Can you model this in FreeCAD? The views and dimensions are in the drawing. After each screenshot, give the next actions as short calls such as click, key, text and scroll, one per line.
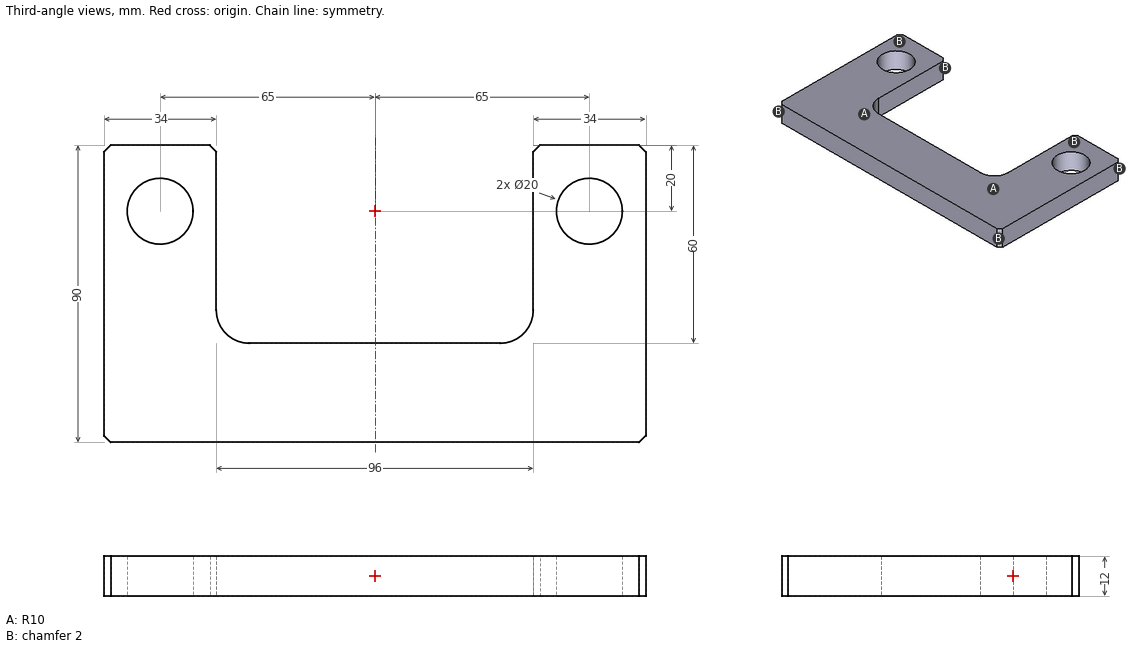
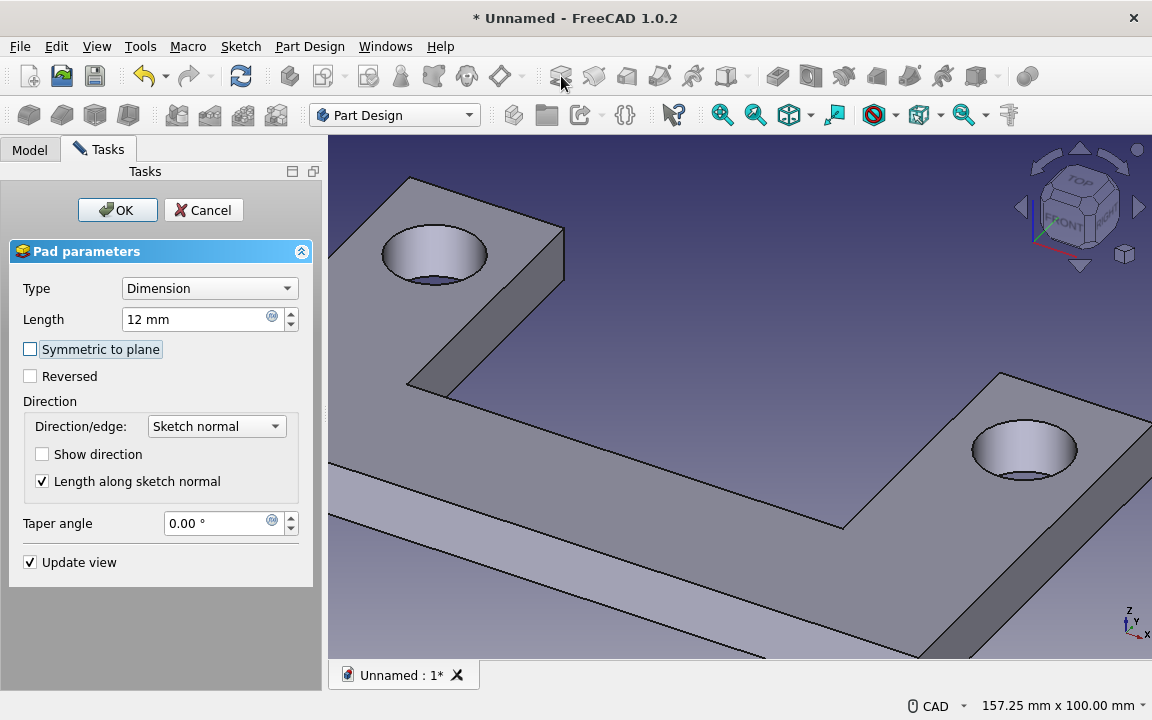
click(31, 349)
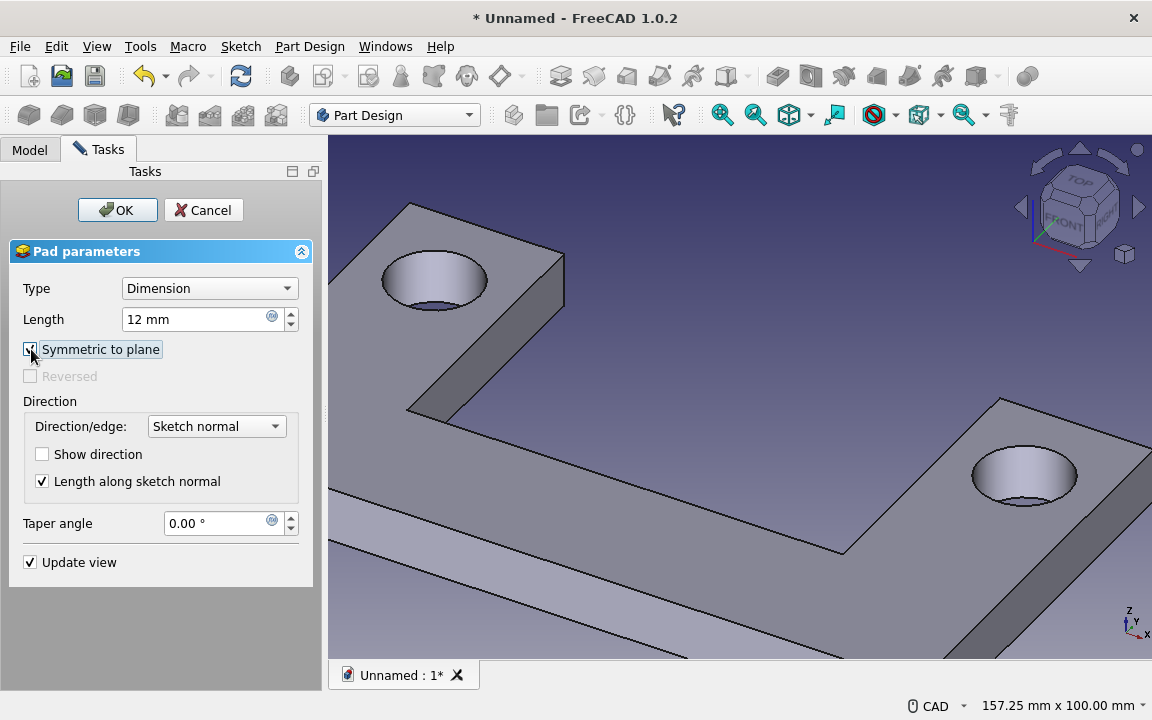
click(118, 210)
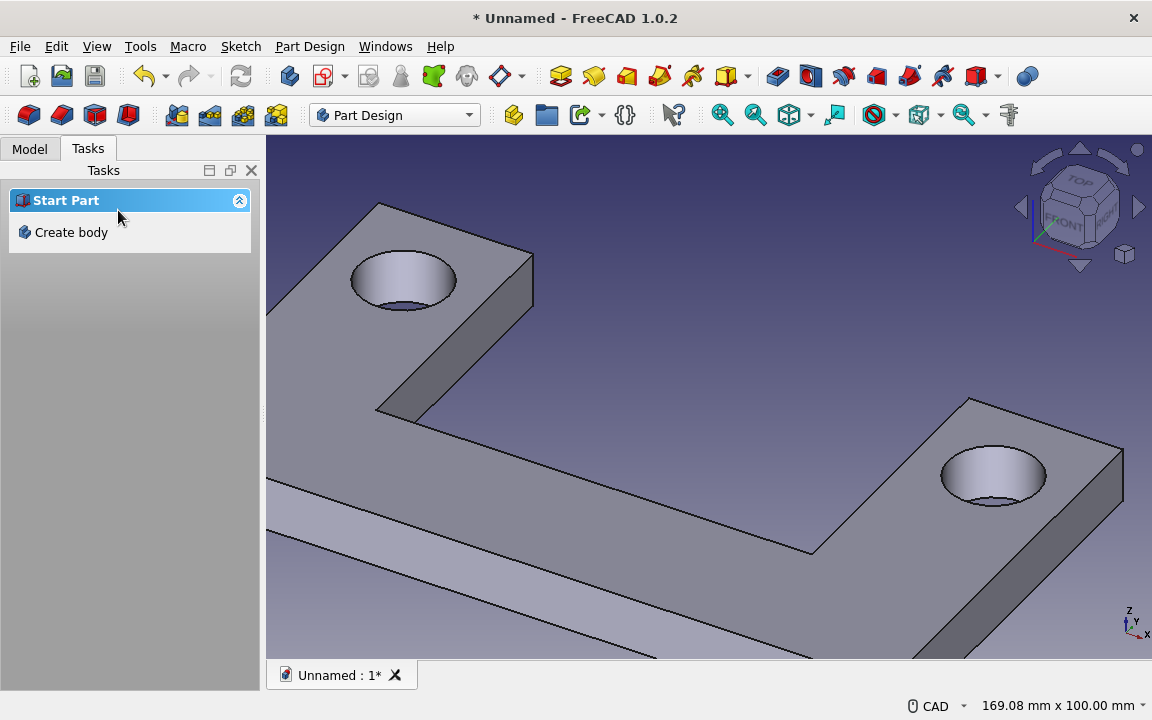
click(723, 116)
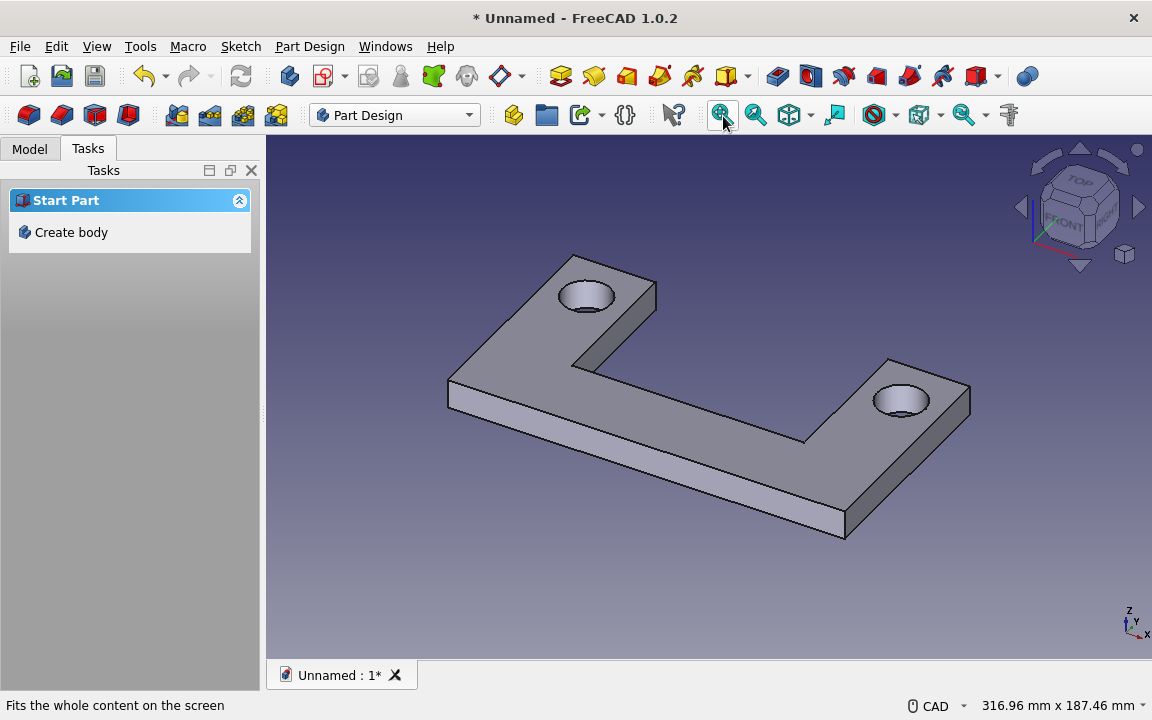
key(0)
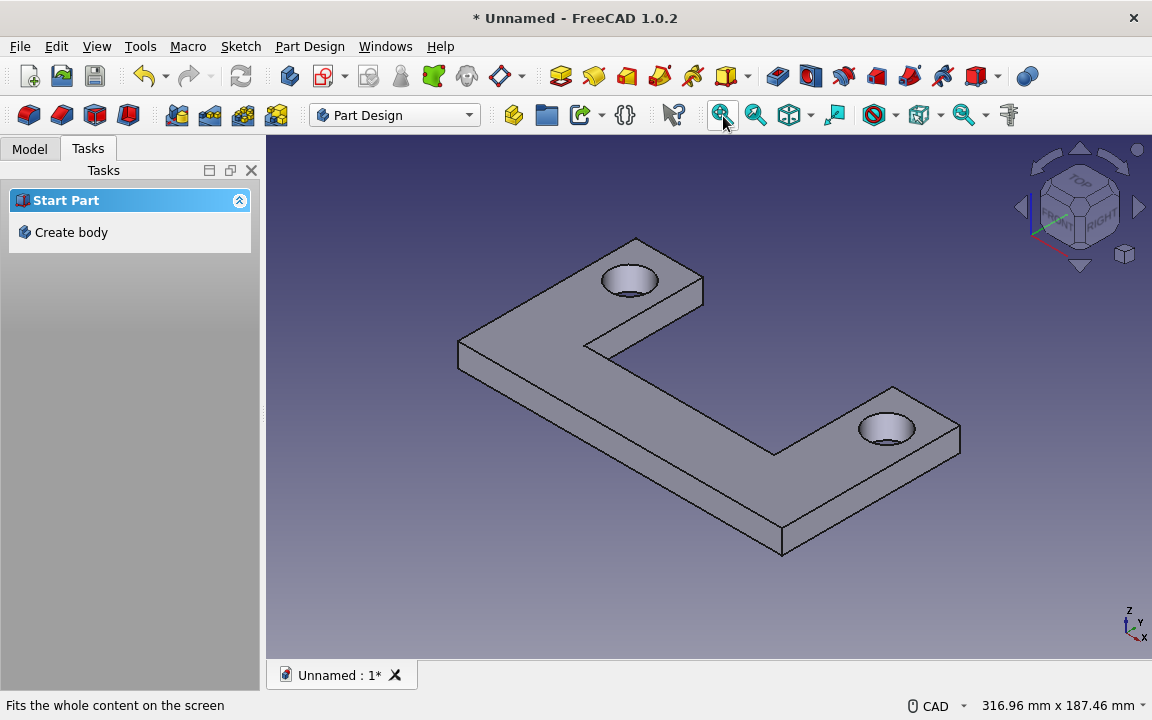
key(2)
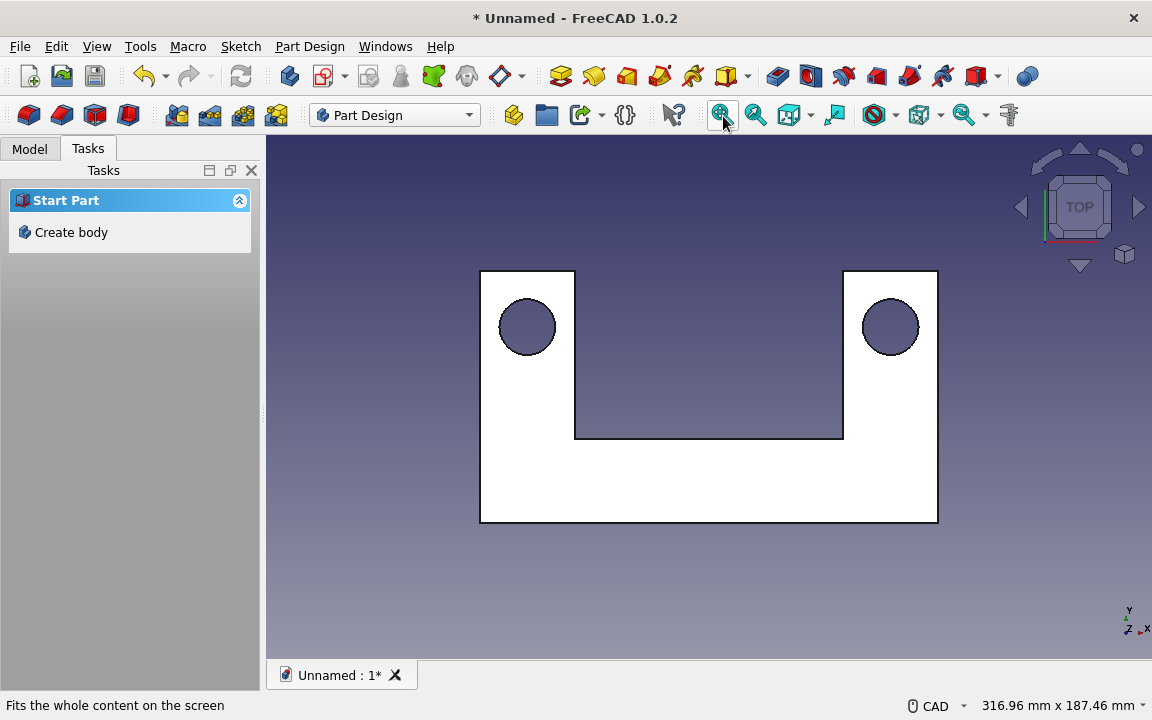
key(1)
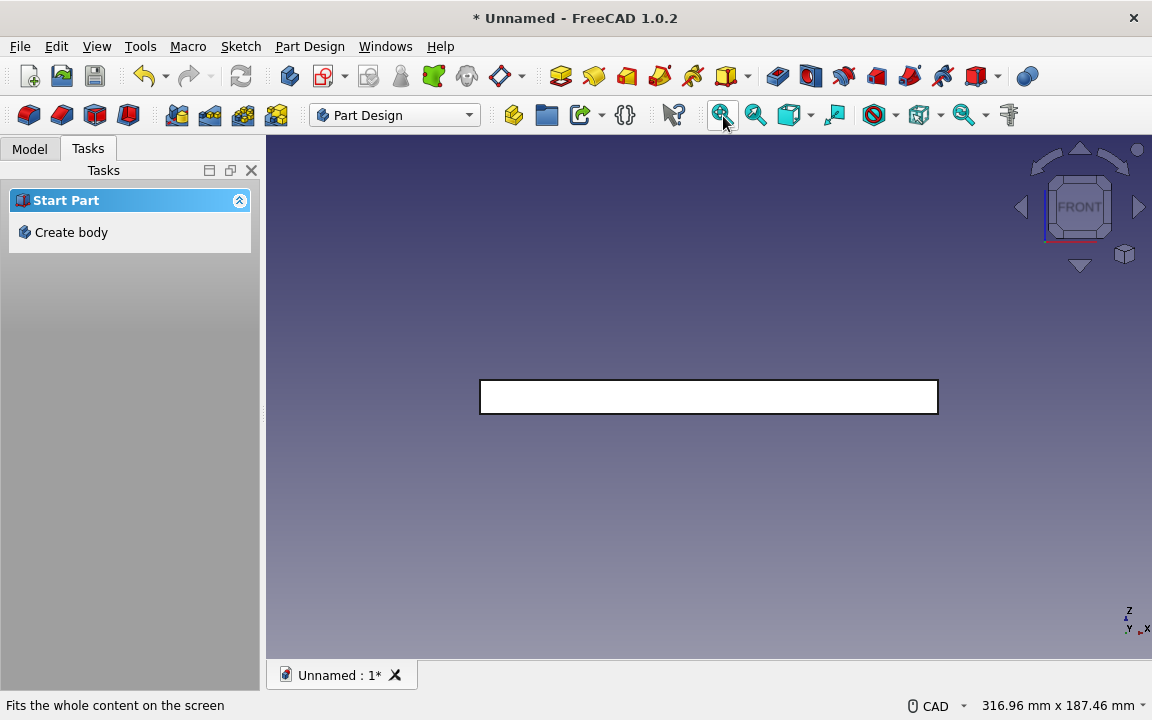
key(3)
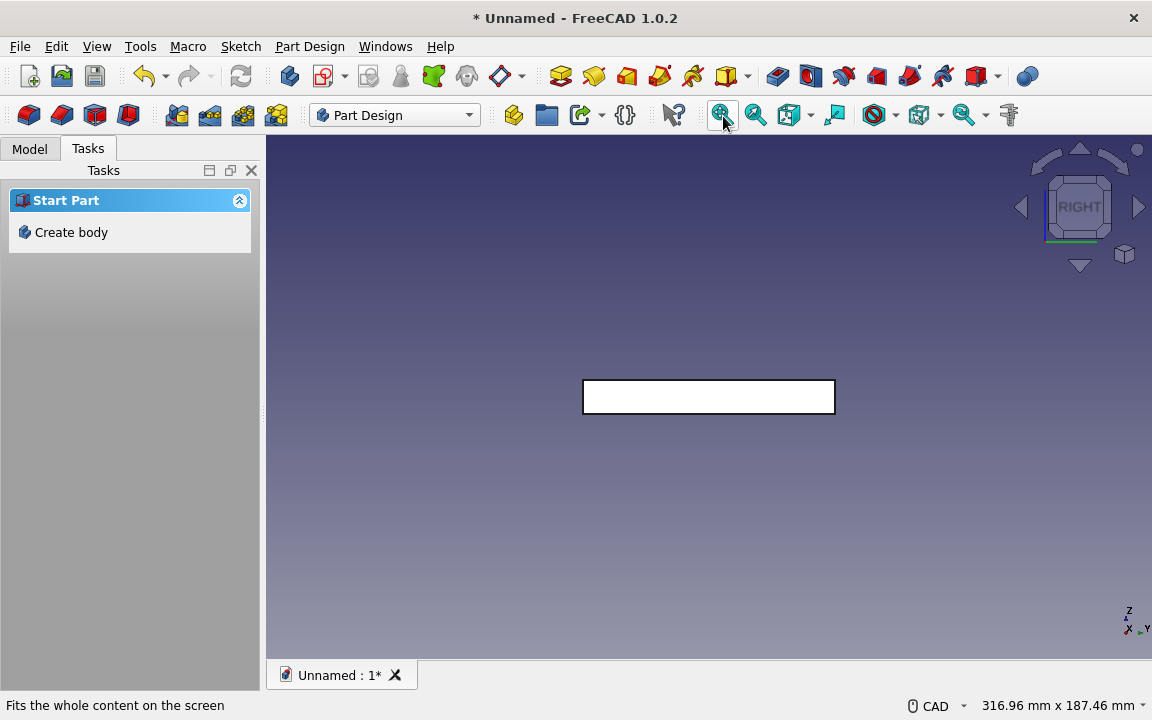
click(723, 116)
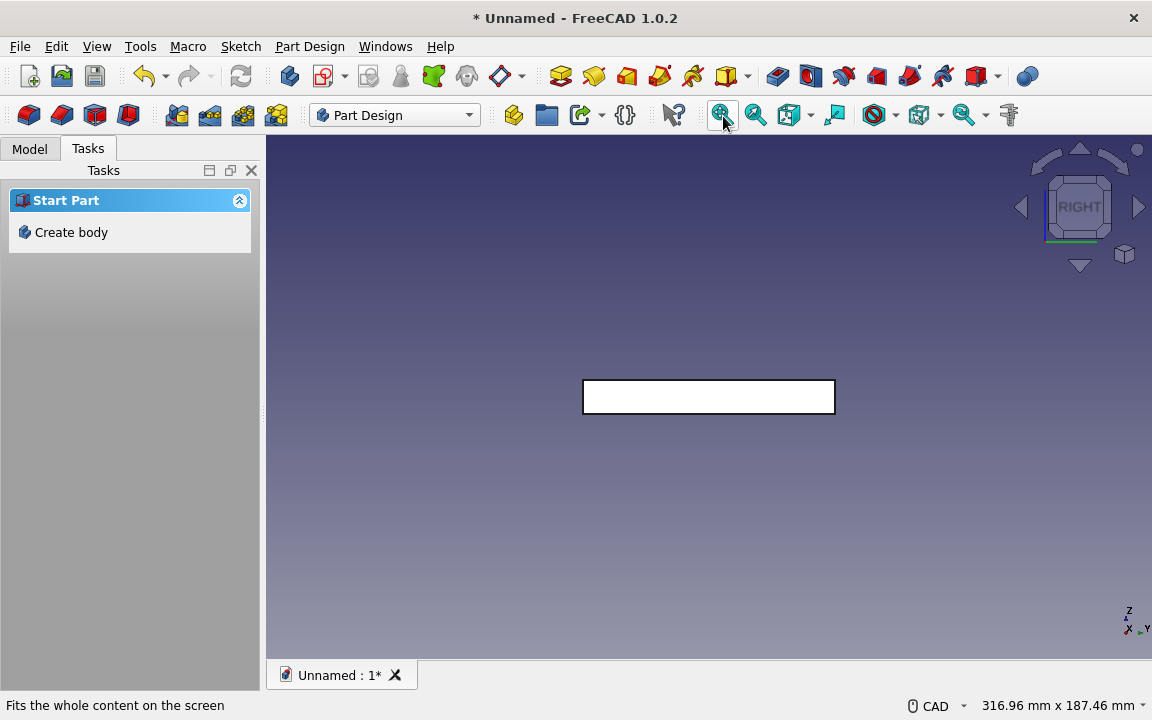
key(5)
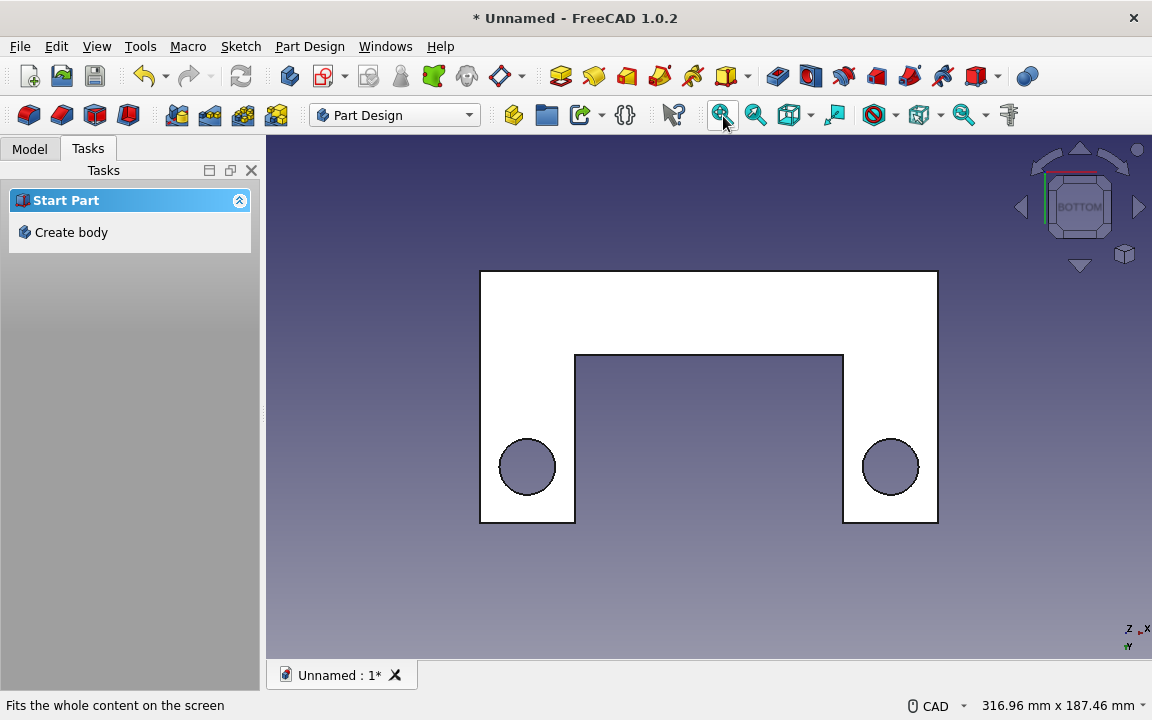
key(4)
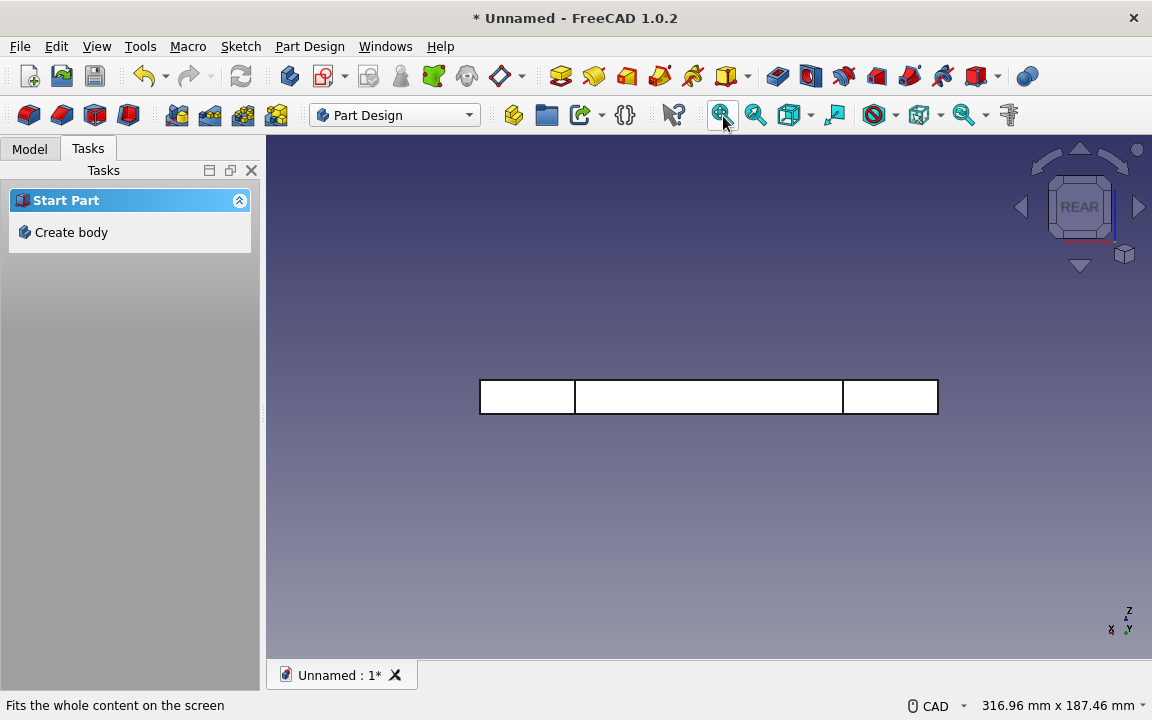
key(6)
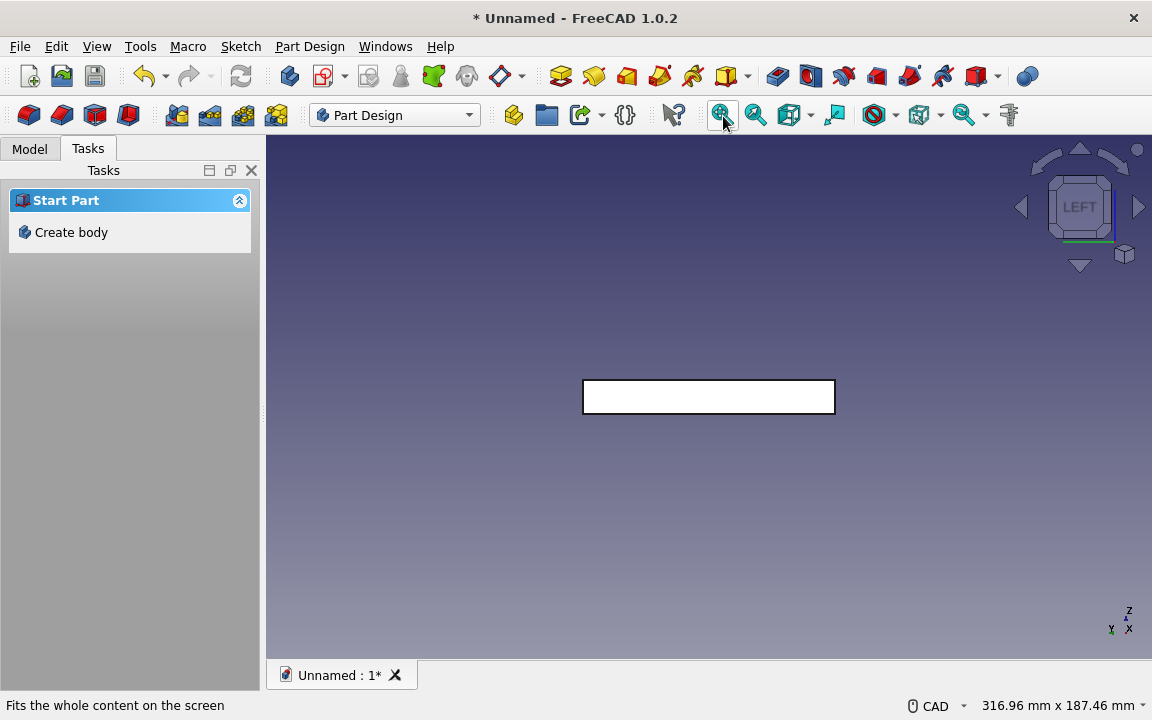
click(723, 116)